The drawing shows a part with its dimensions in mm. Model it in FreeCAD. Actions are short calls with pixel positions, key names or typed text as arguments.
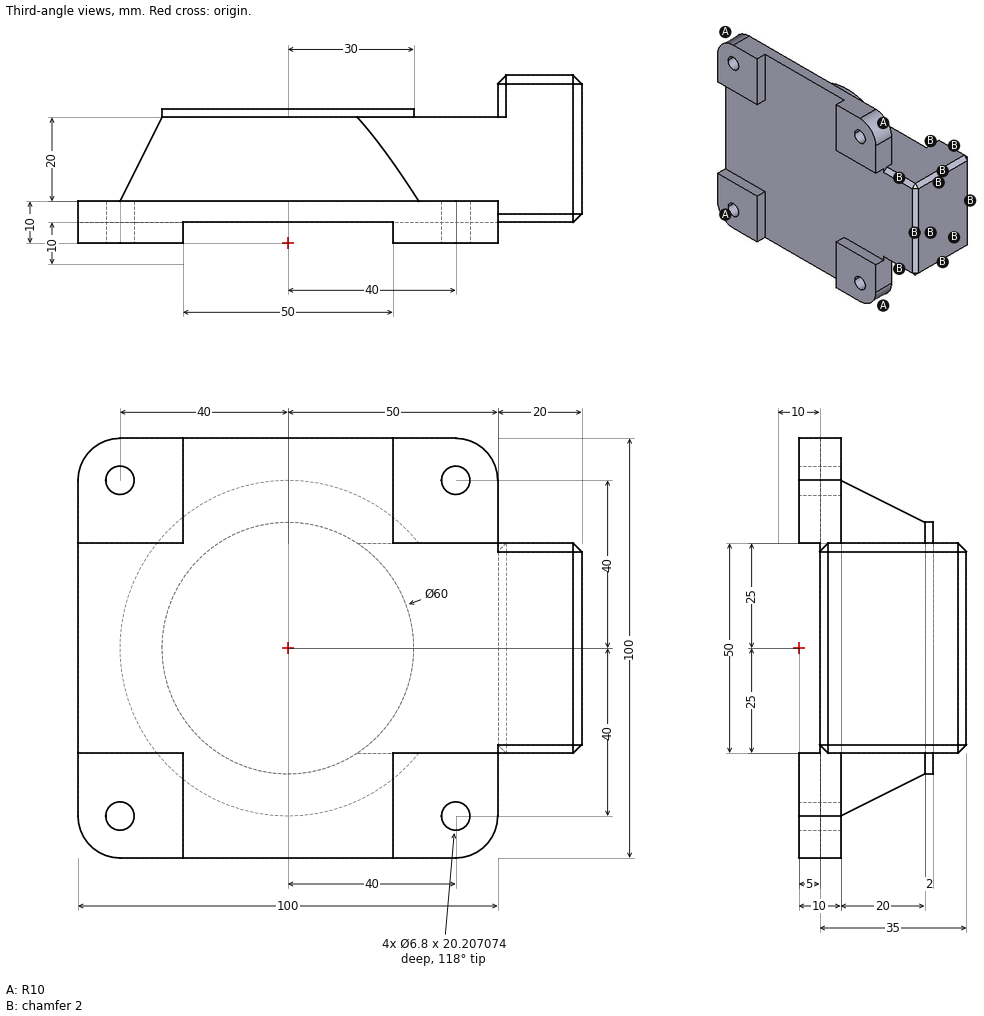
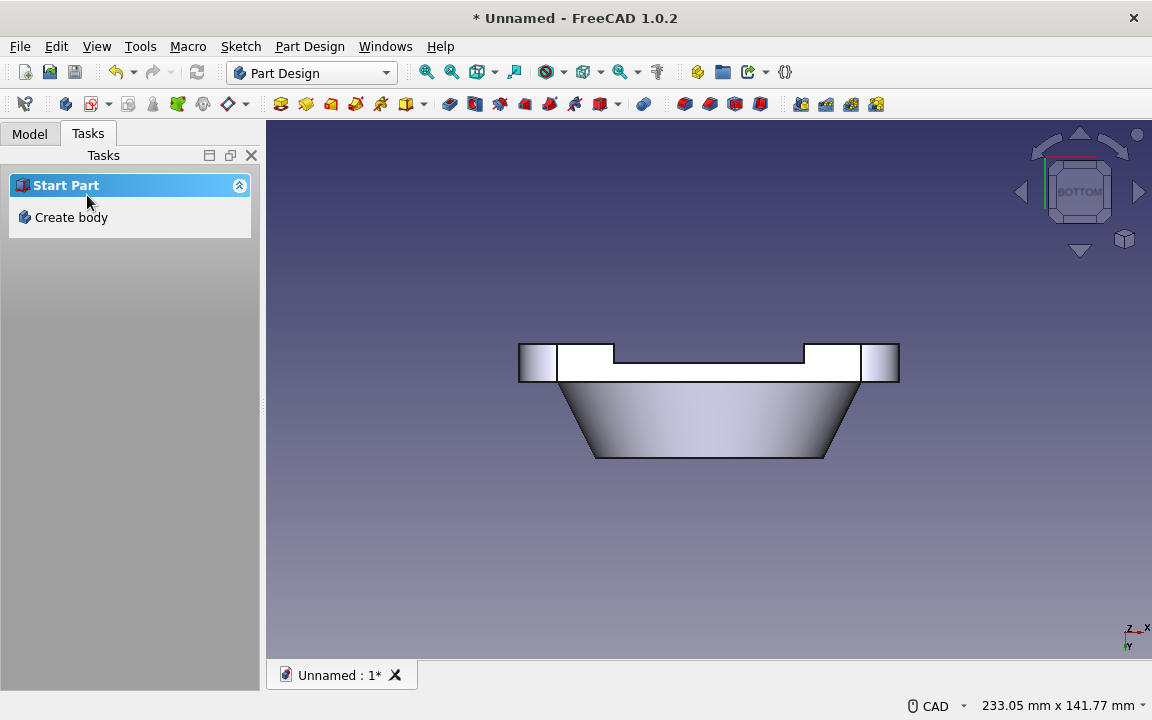
click(427, 72)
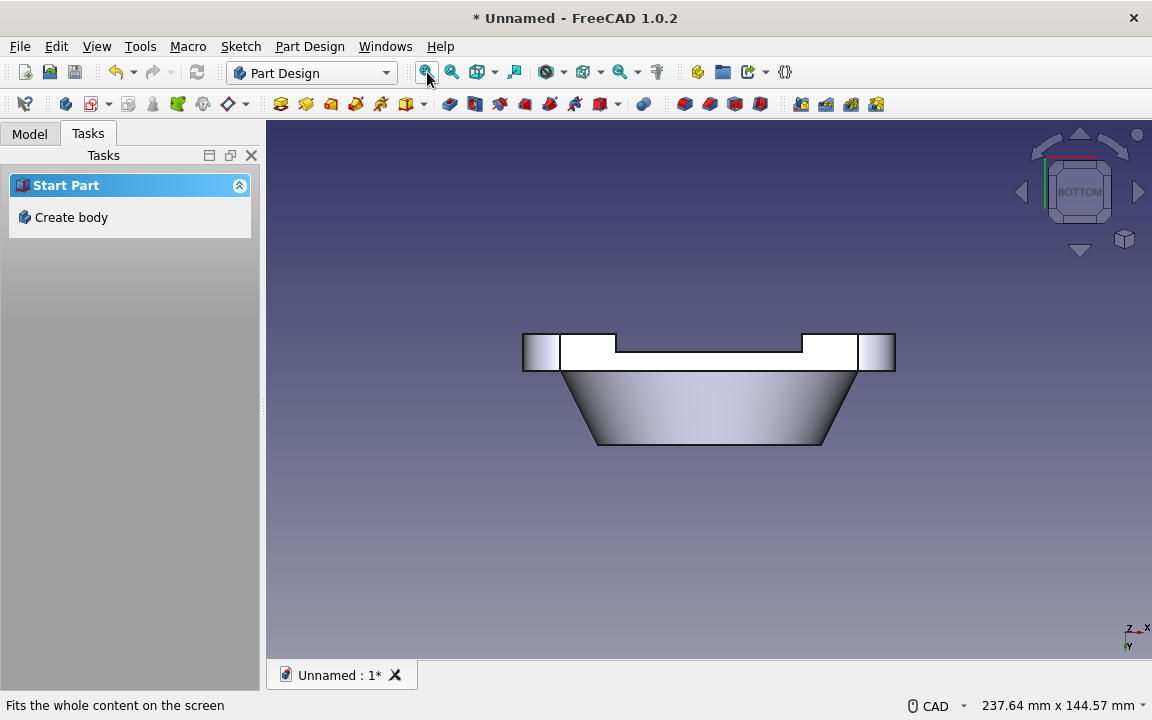
key(4)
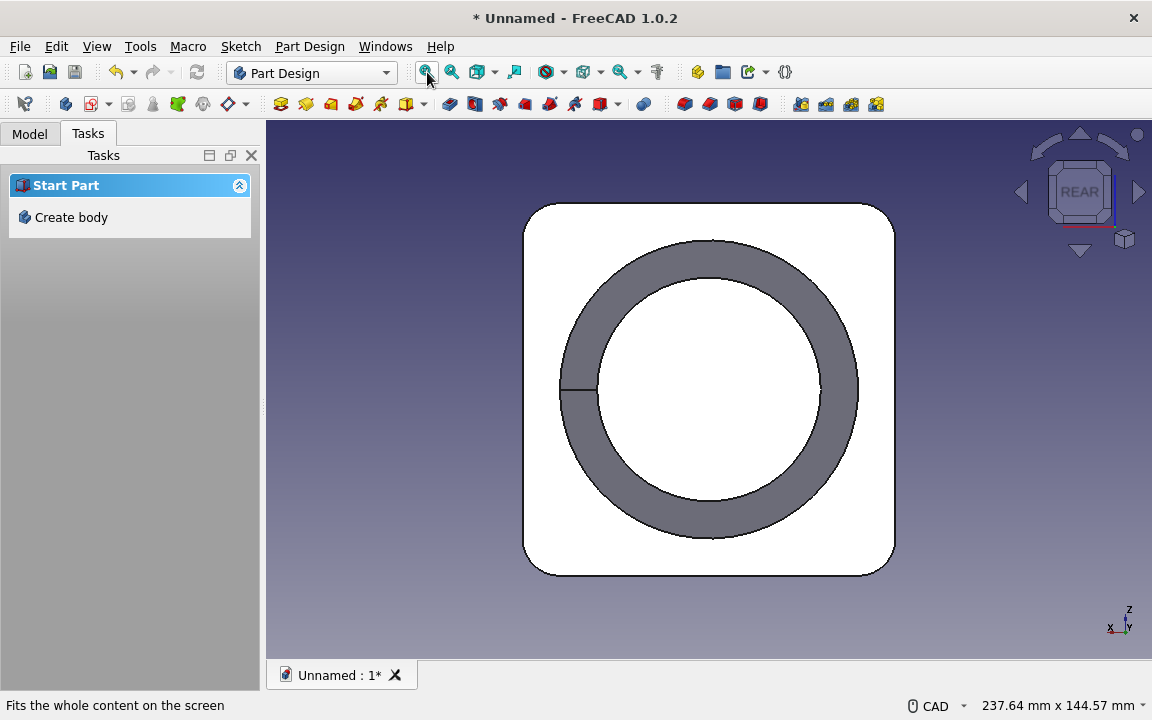
click(709, 388)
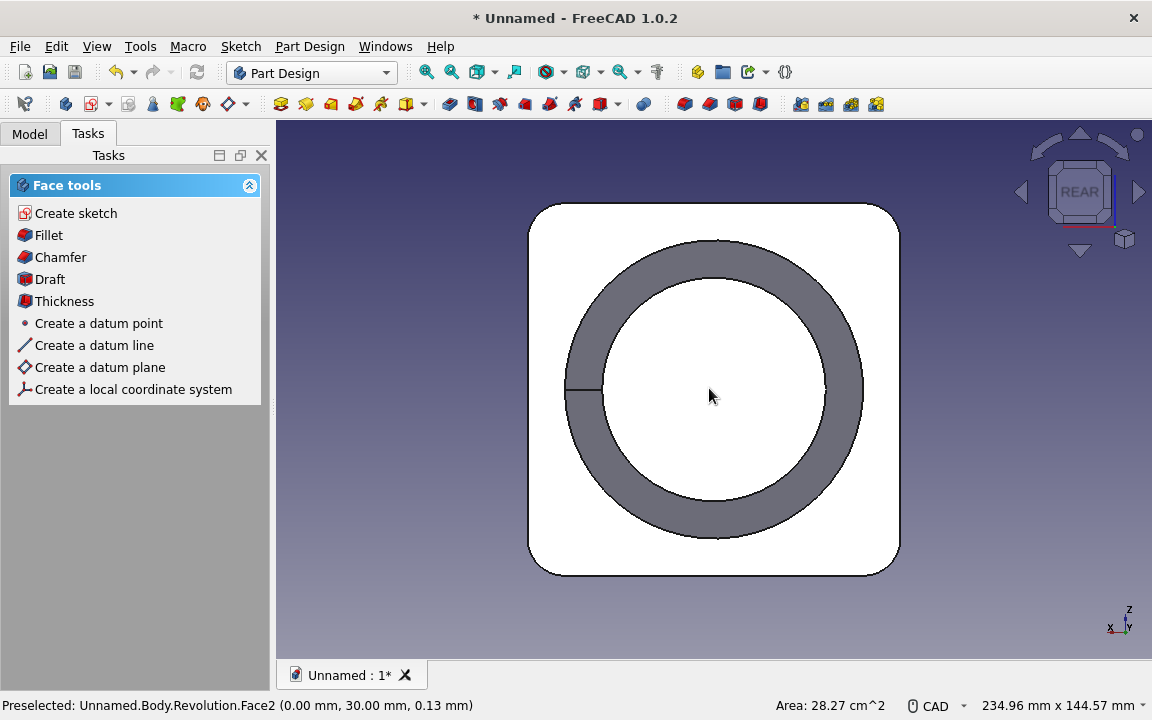
click(90, 104)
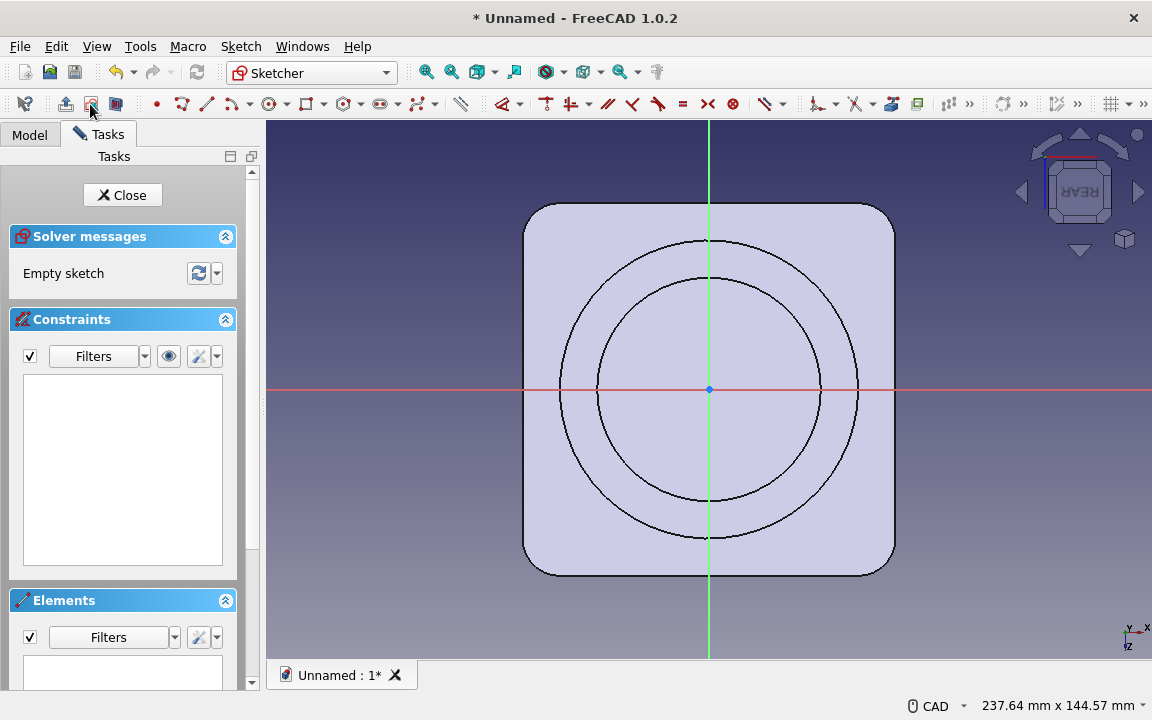
scroll(848, 390, up, 2)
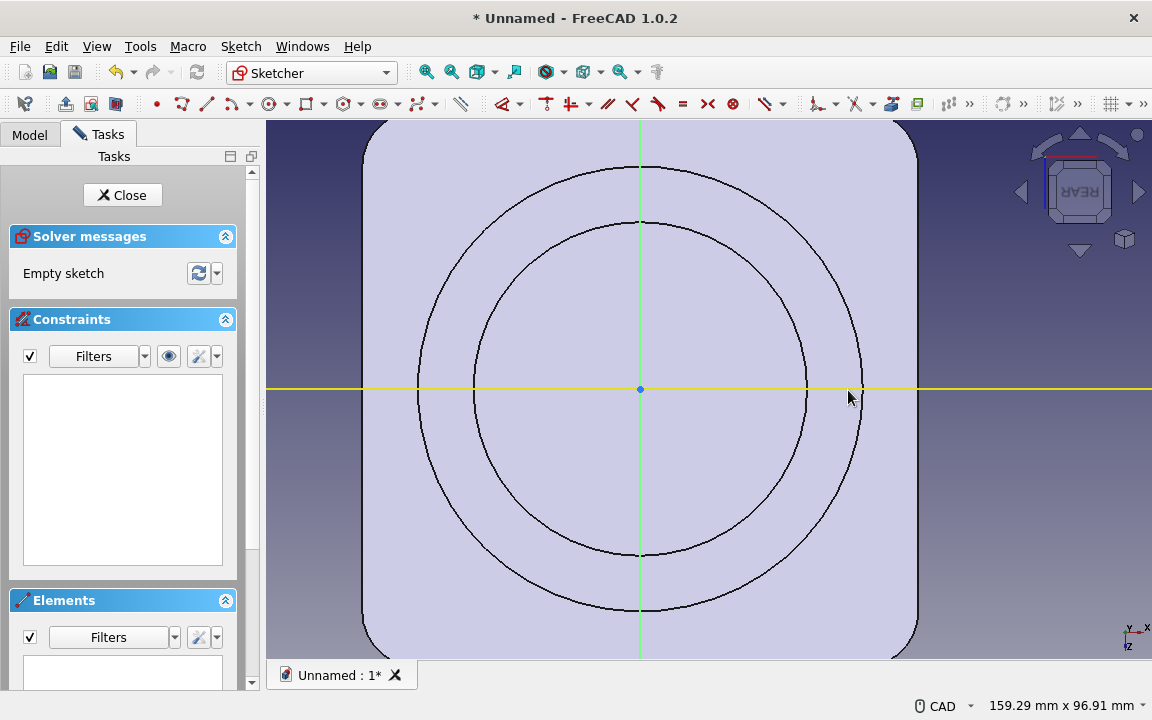
click(268, 104)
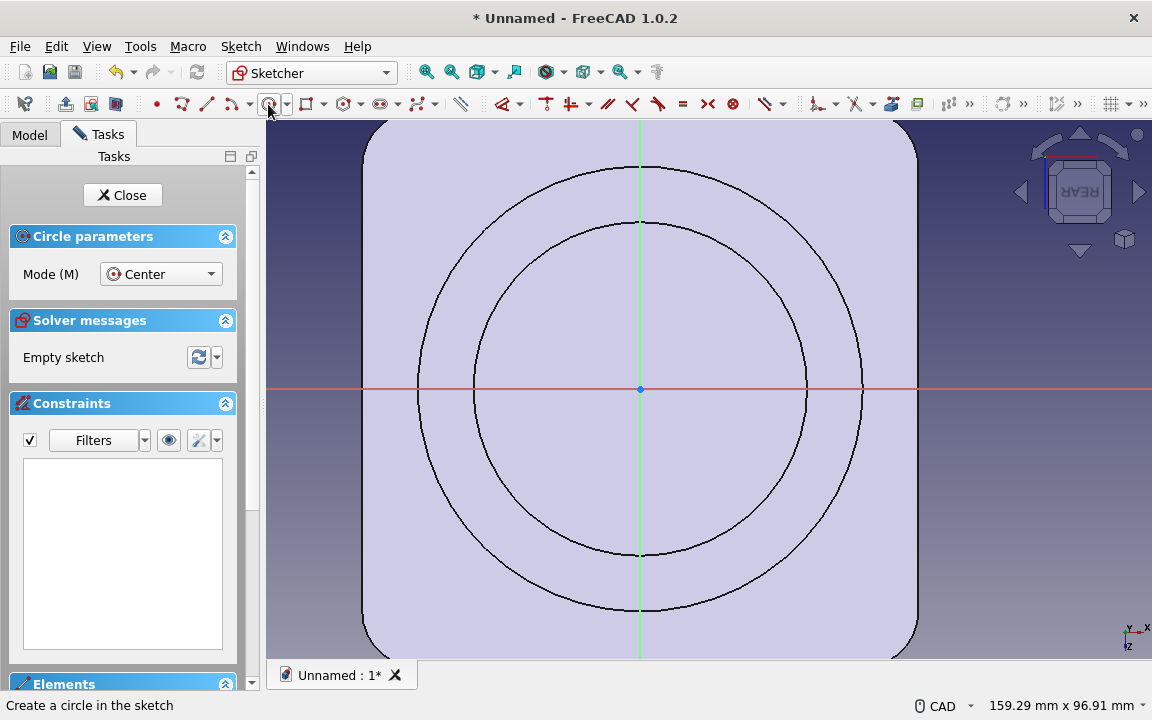
click(640, 389)
click(758, 271)
key(Escape)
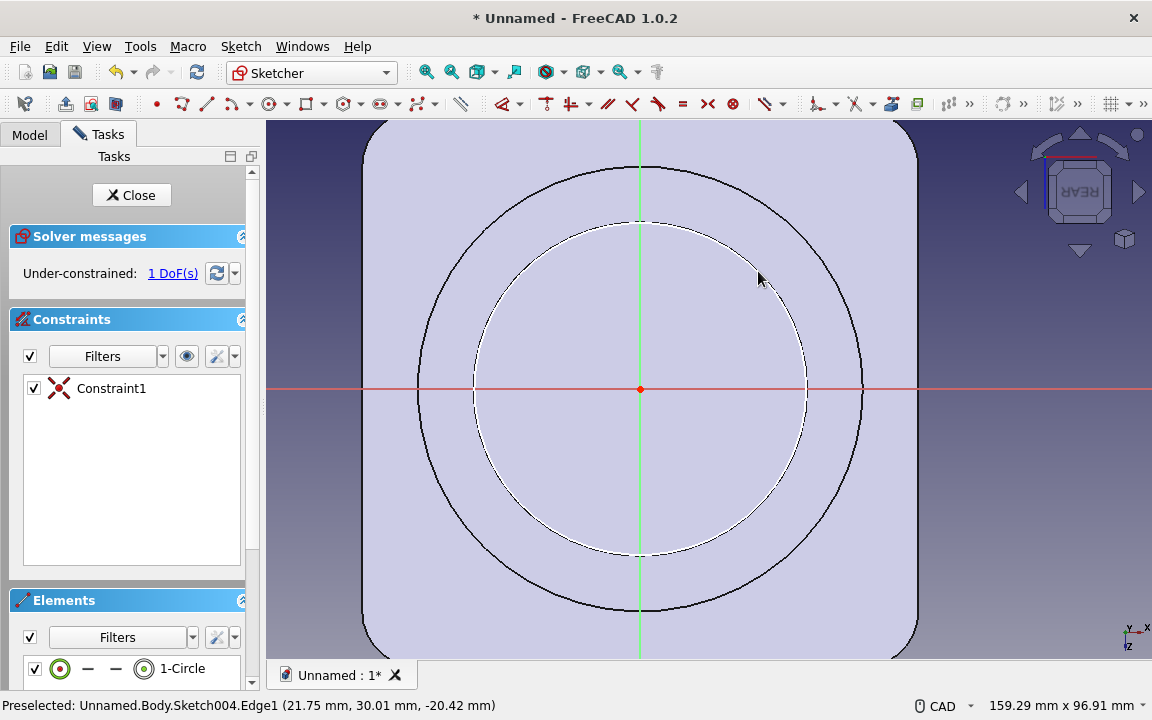
click(502, 104)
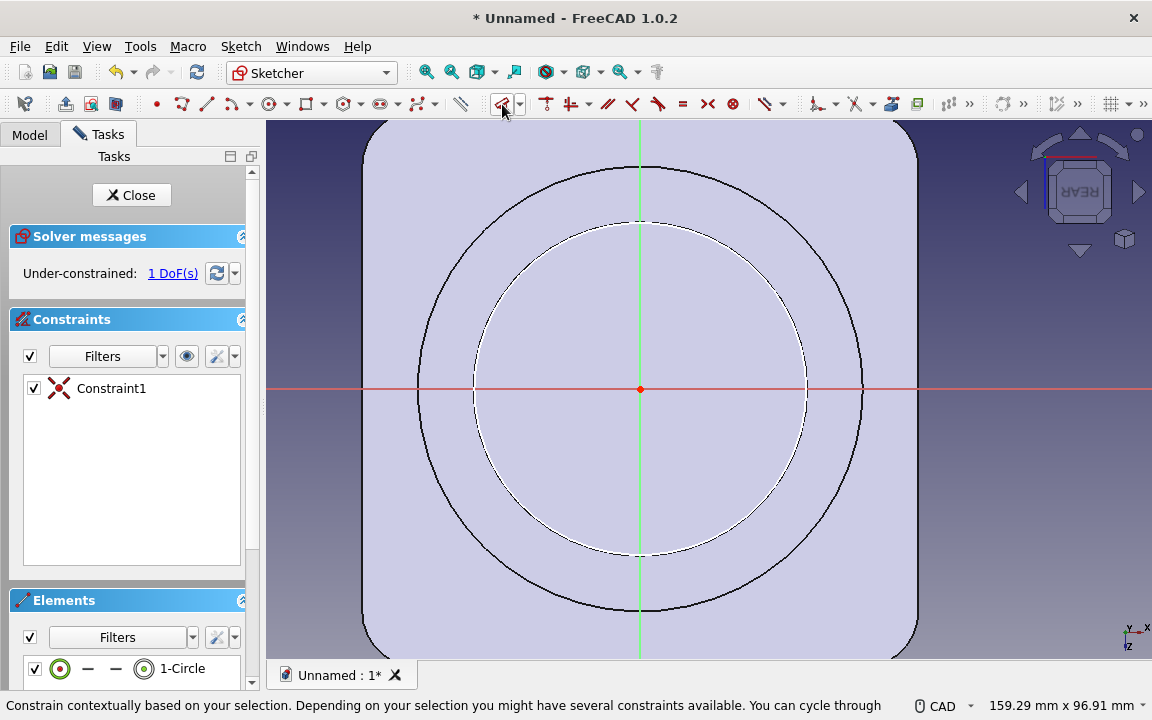
click(757, 271)
click(779, 248)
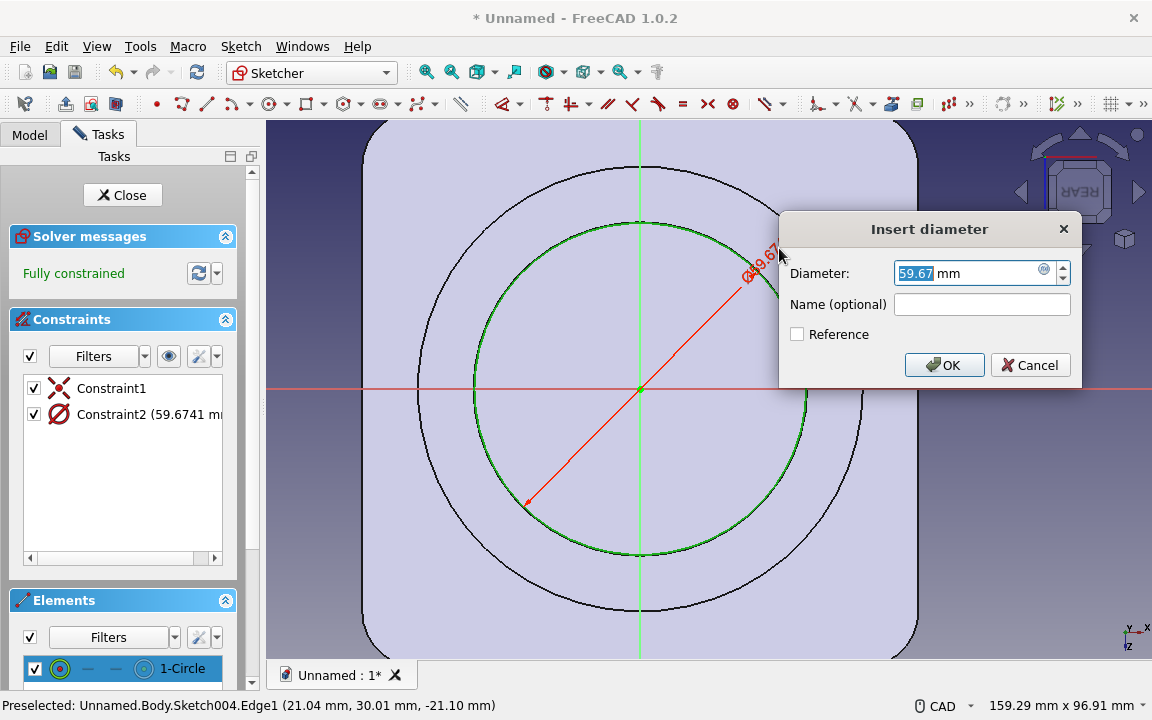
text(60)
key(Return)
key(Escape)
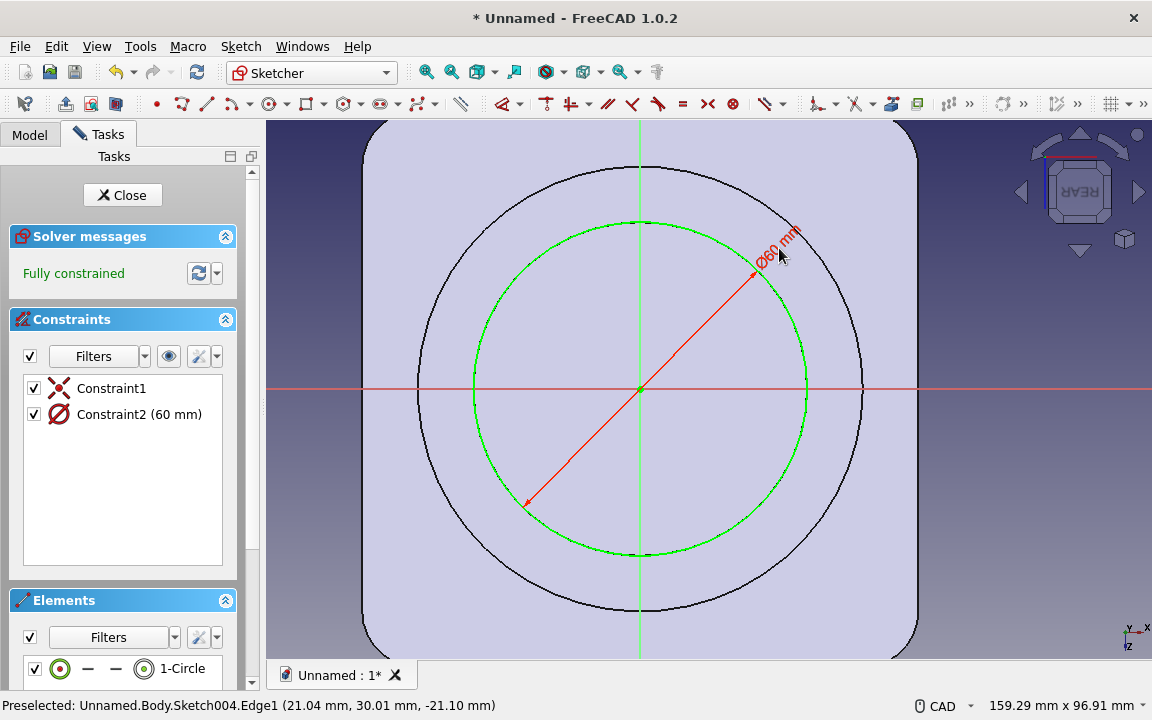
click(123, 195)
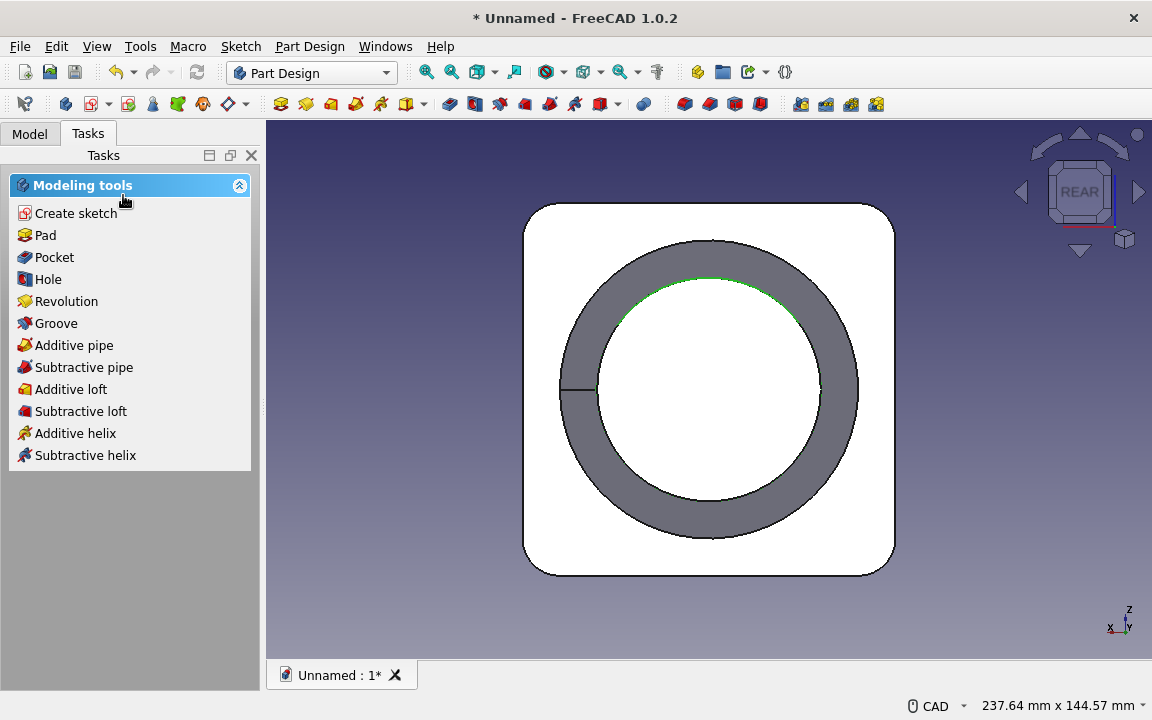
click(281, 104)